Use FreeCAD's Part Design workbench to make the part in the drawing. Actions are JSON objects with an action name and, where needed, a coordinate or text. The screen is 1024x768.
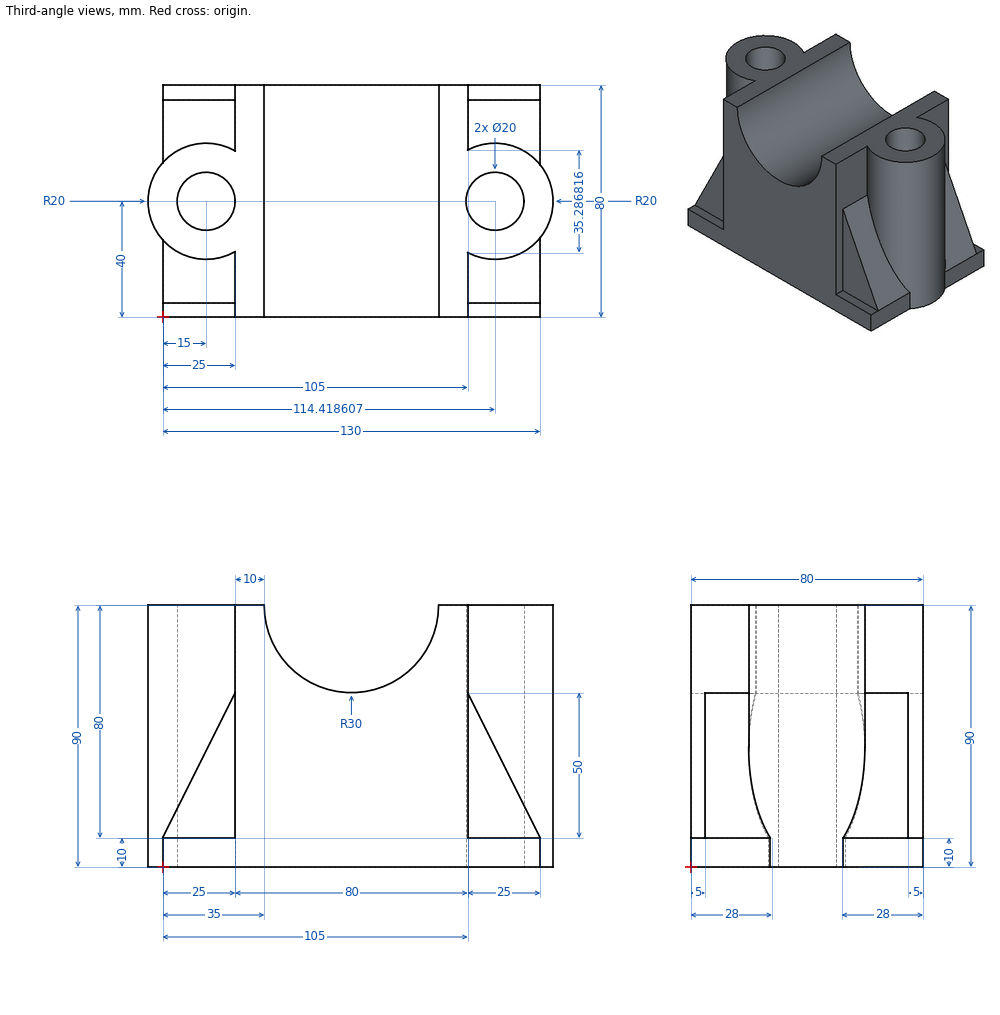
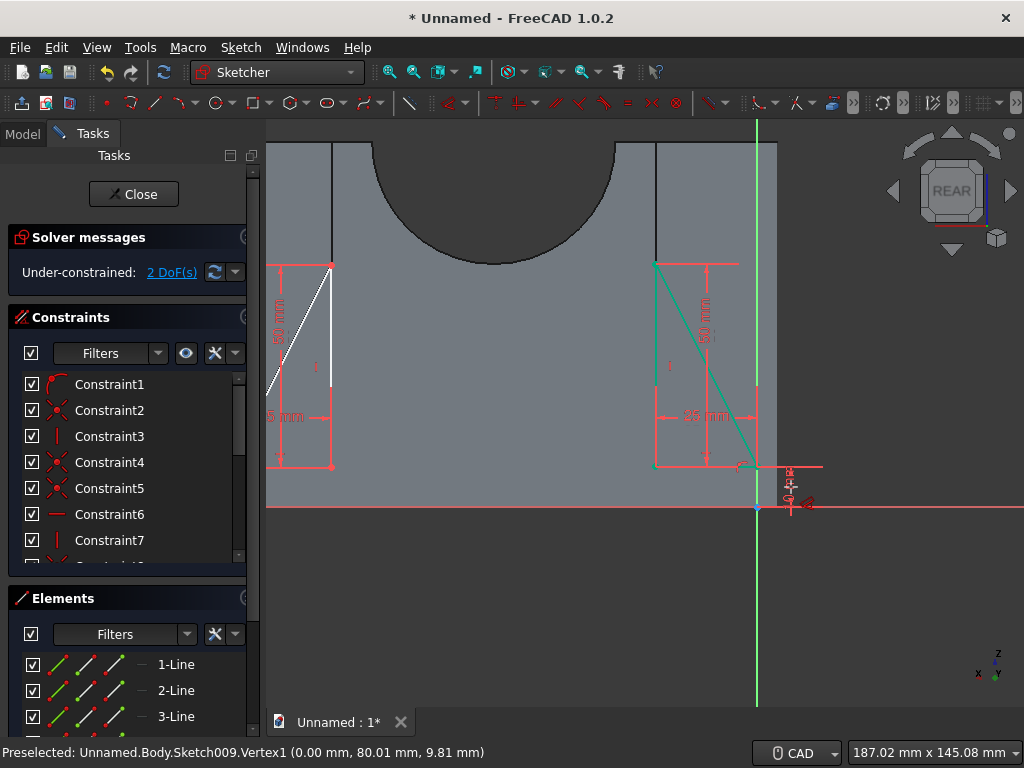
{"action": "left_click", "coordinate": [331, 468]}
{"action": "left_click", "coordinate": [297, 487]}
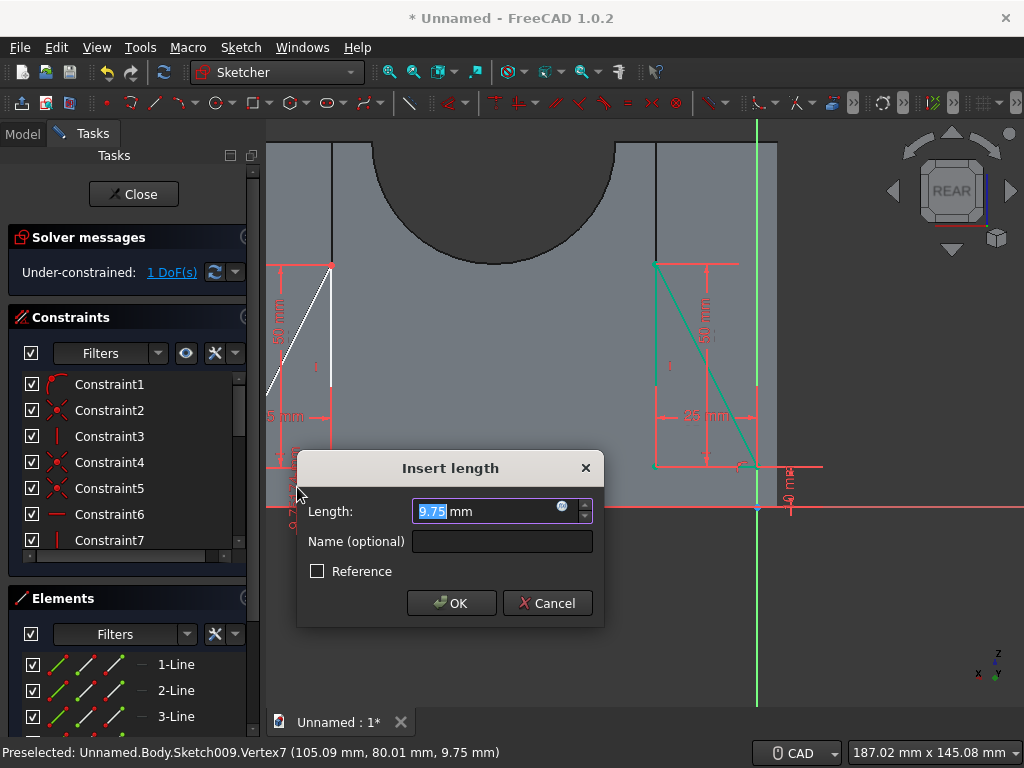
{"action": "type", "text": "10"}
{"action": "key", "text": "Return"}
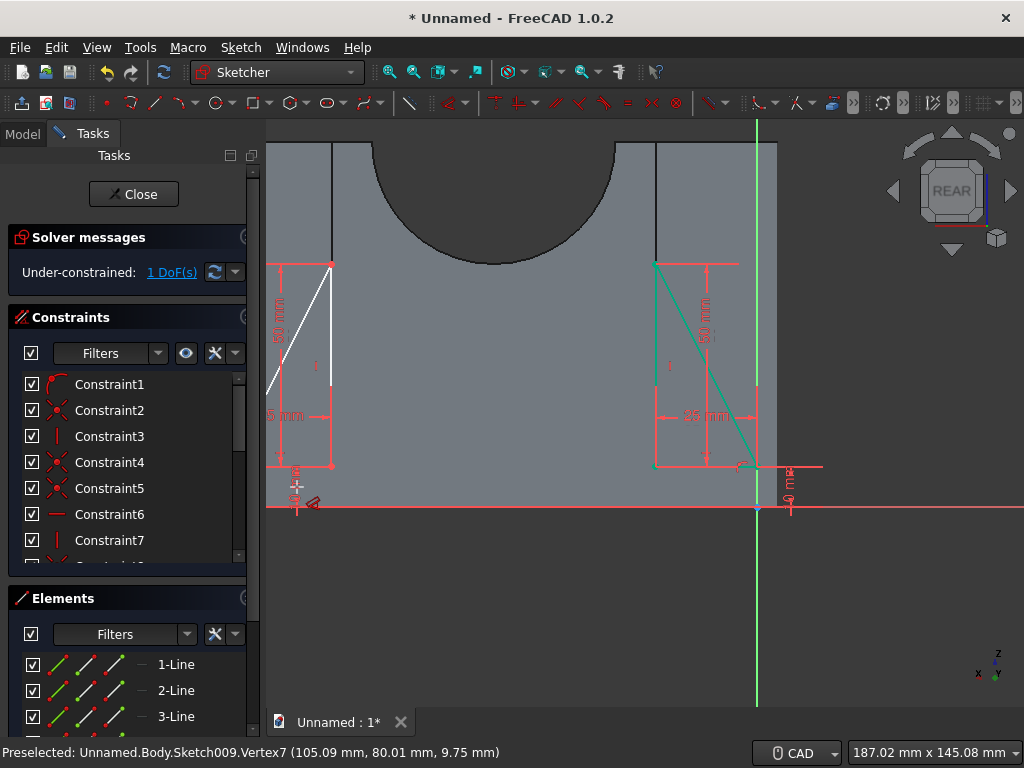
{"action": "left_click", "coordinate": [331, 467]}
{"action": "left_click", "coordinate": [544, 541]}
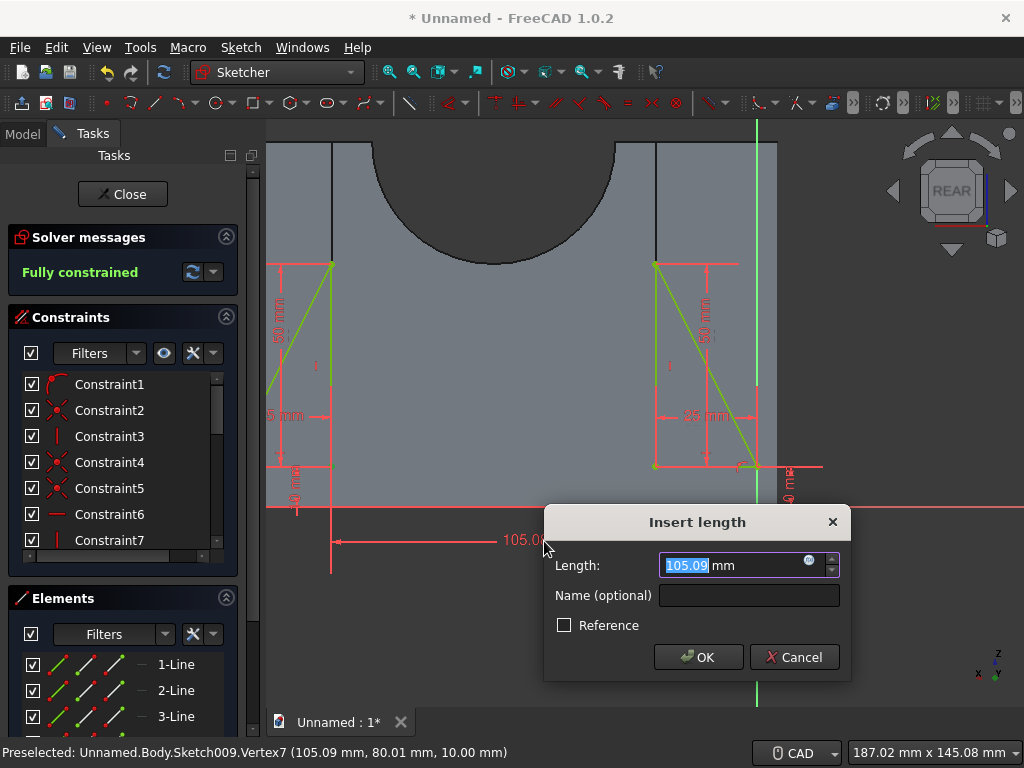
{"action": "type", "text": "105"}
{"action": "key", "text": "Return"}
{"action": "key", "text": "Escape"}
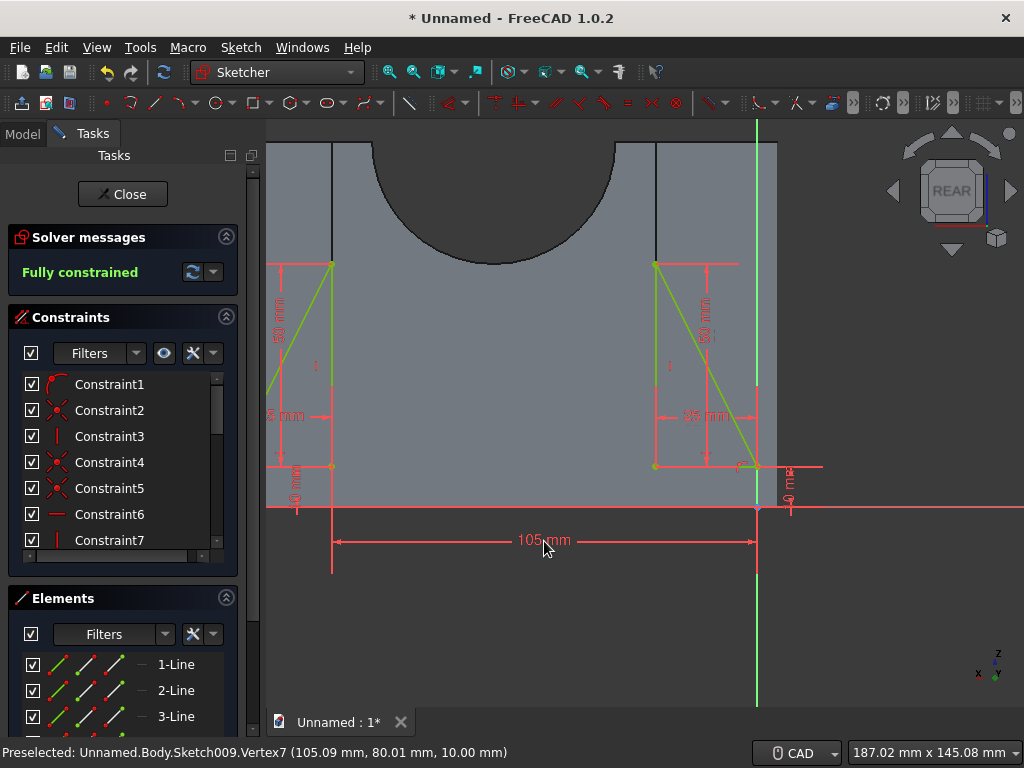
{"action": "left_click", "coordinate": [123, 194]}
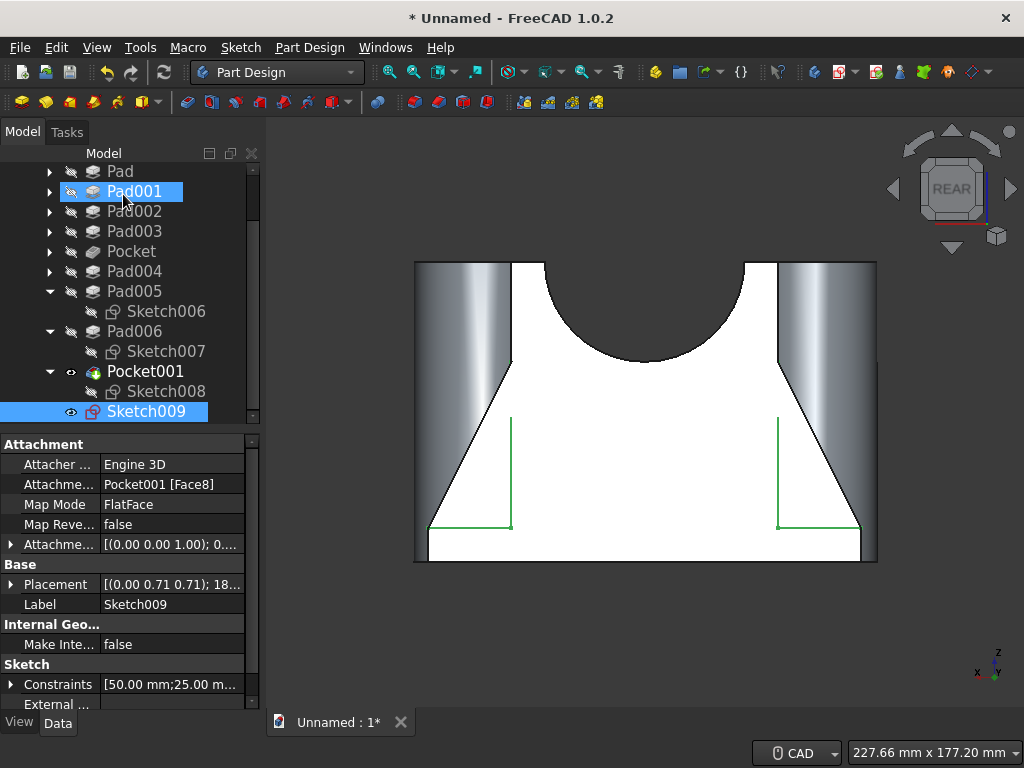
{"action": "left_click", "coordinate": [188, 102]}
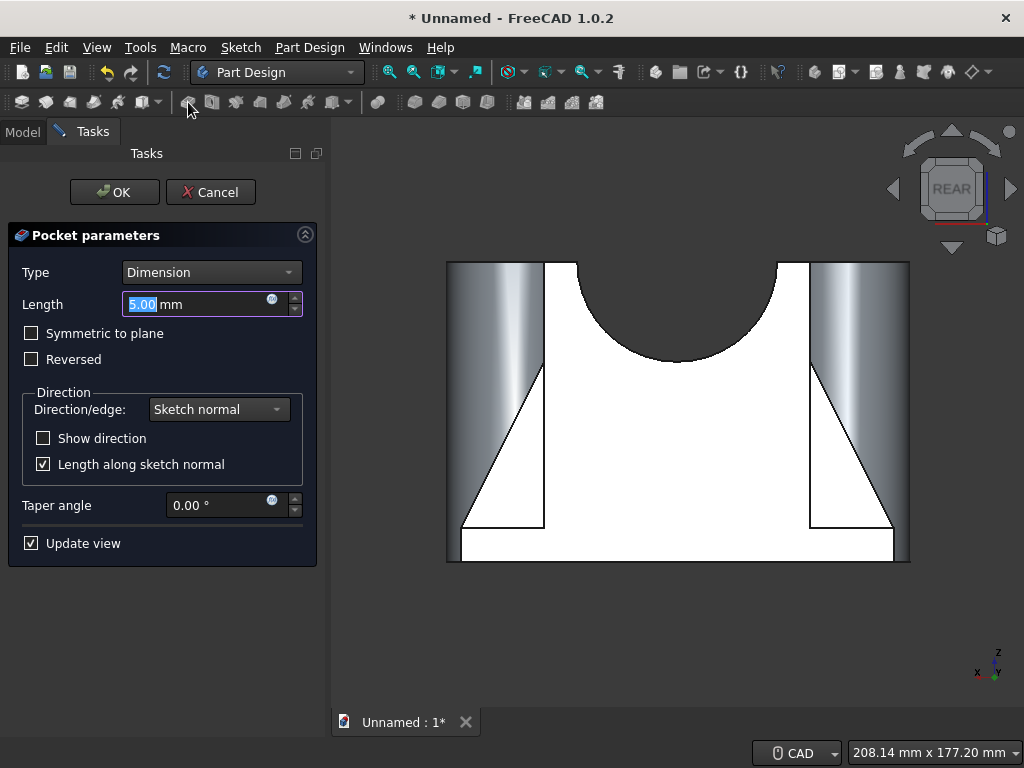
{"action": "type", "text": "5"}
{"action": "key", "text": "Tab"}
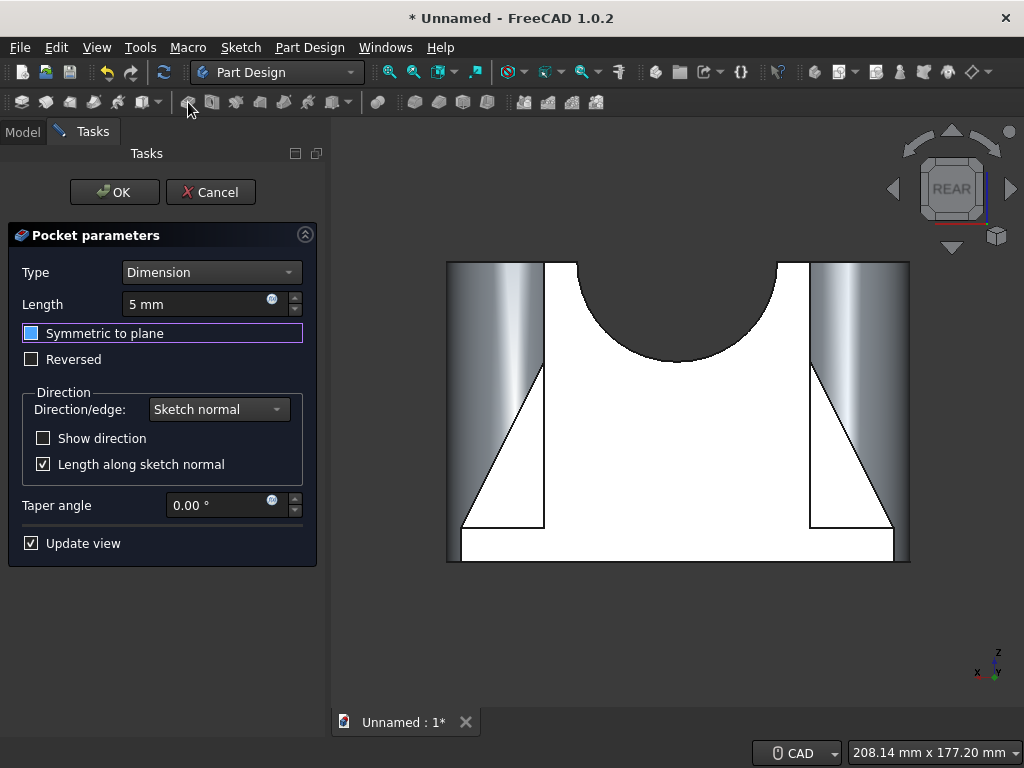
{"action": "left_click", "coordinate": [115, 192]}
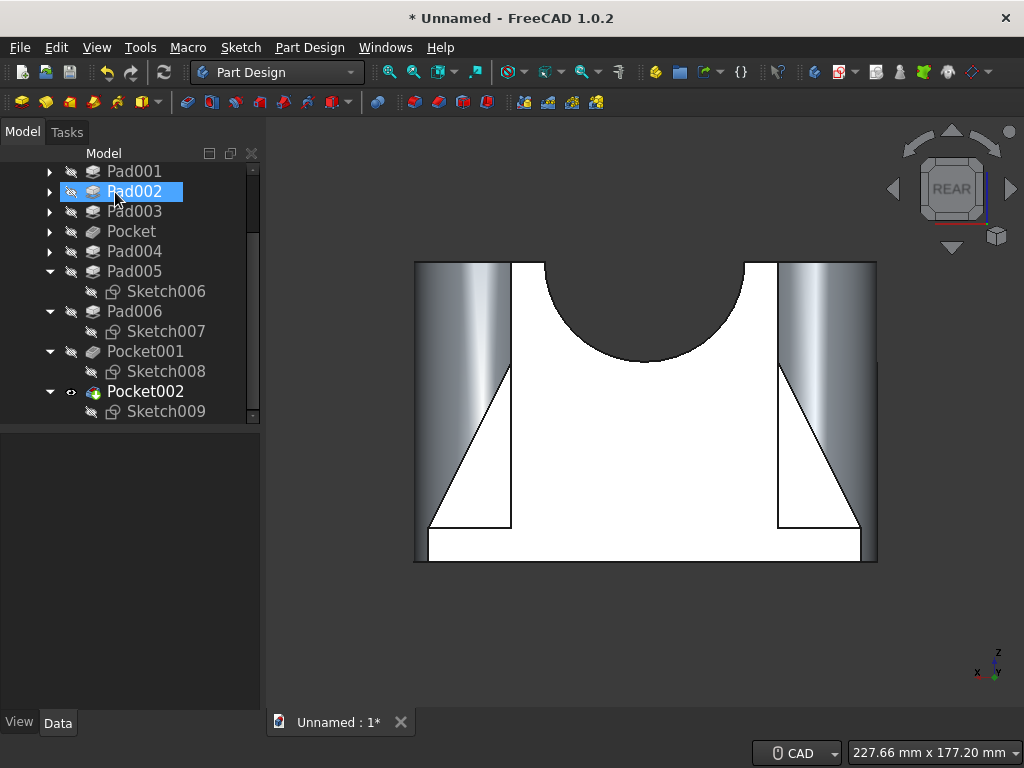
{"action": "key", "text": "0"}